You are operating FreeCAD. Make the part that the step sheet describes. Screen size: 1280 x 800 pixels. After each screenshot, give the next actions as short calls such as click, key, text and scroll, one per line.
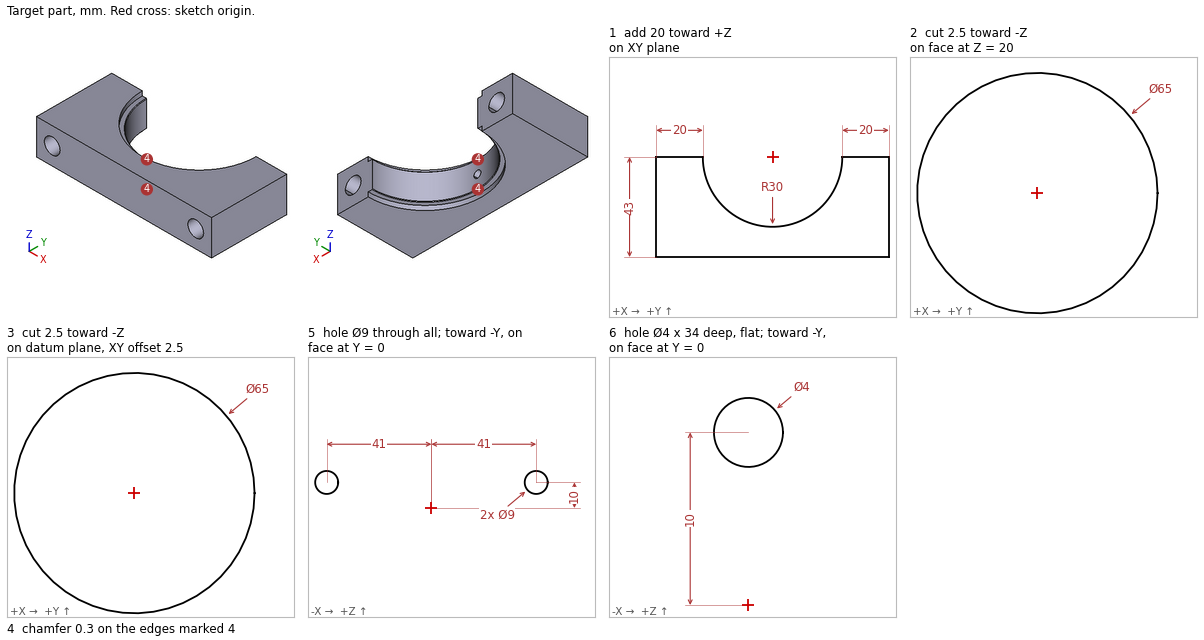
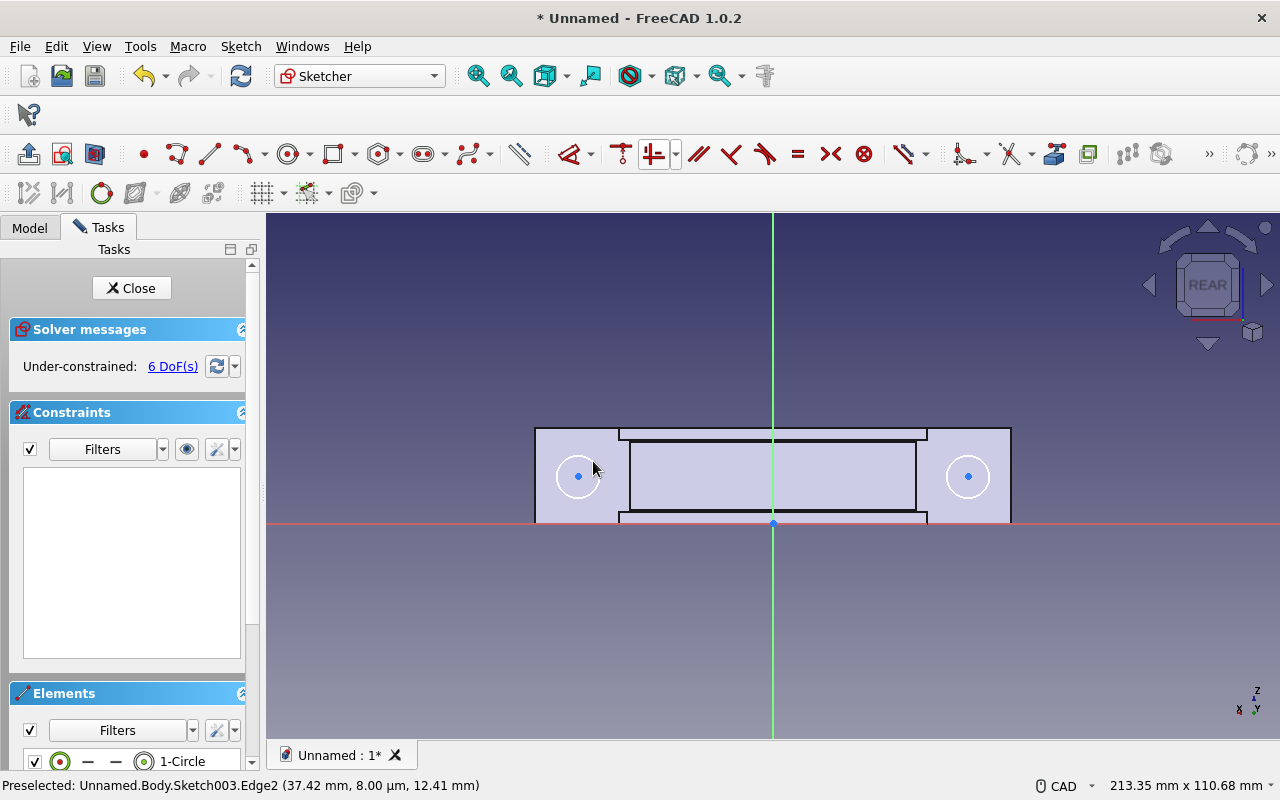
click(983, 462)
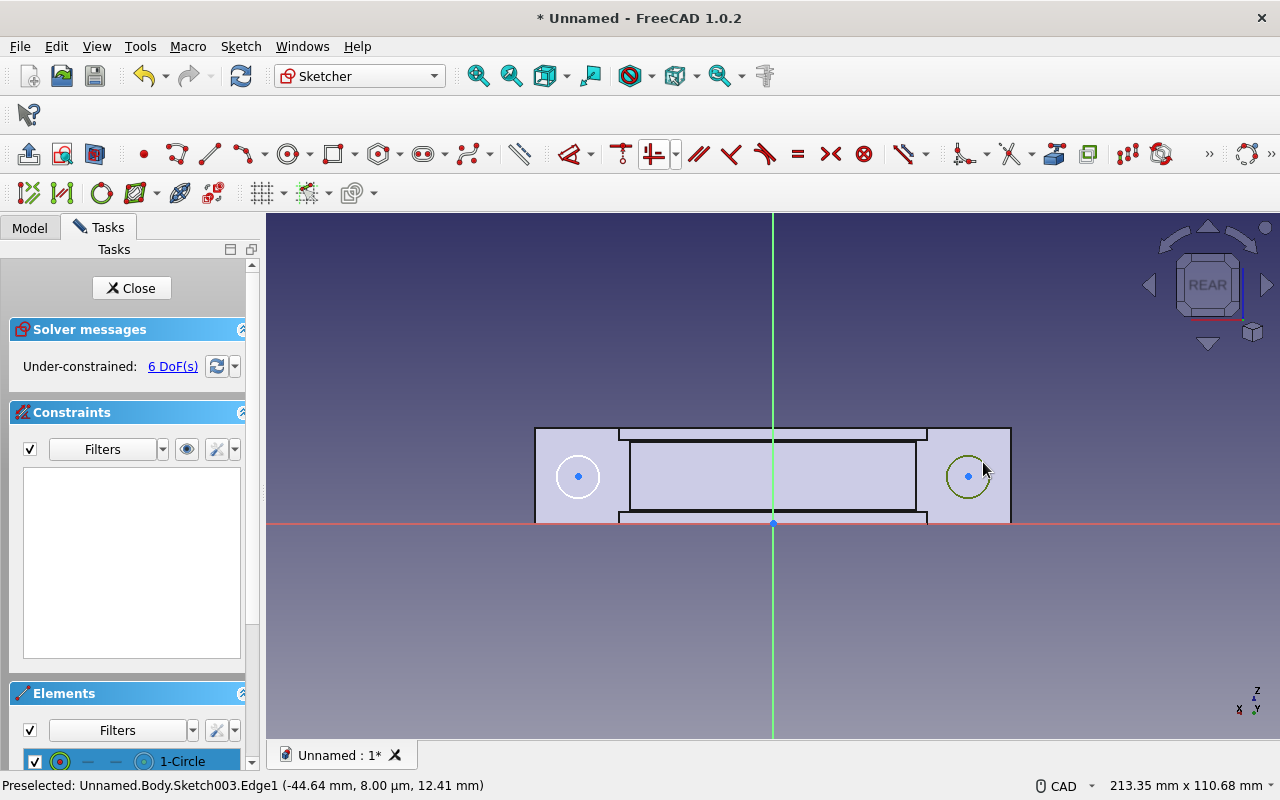
click(593, 462)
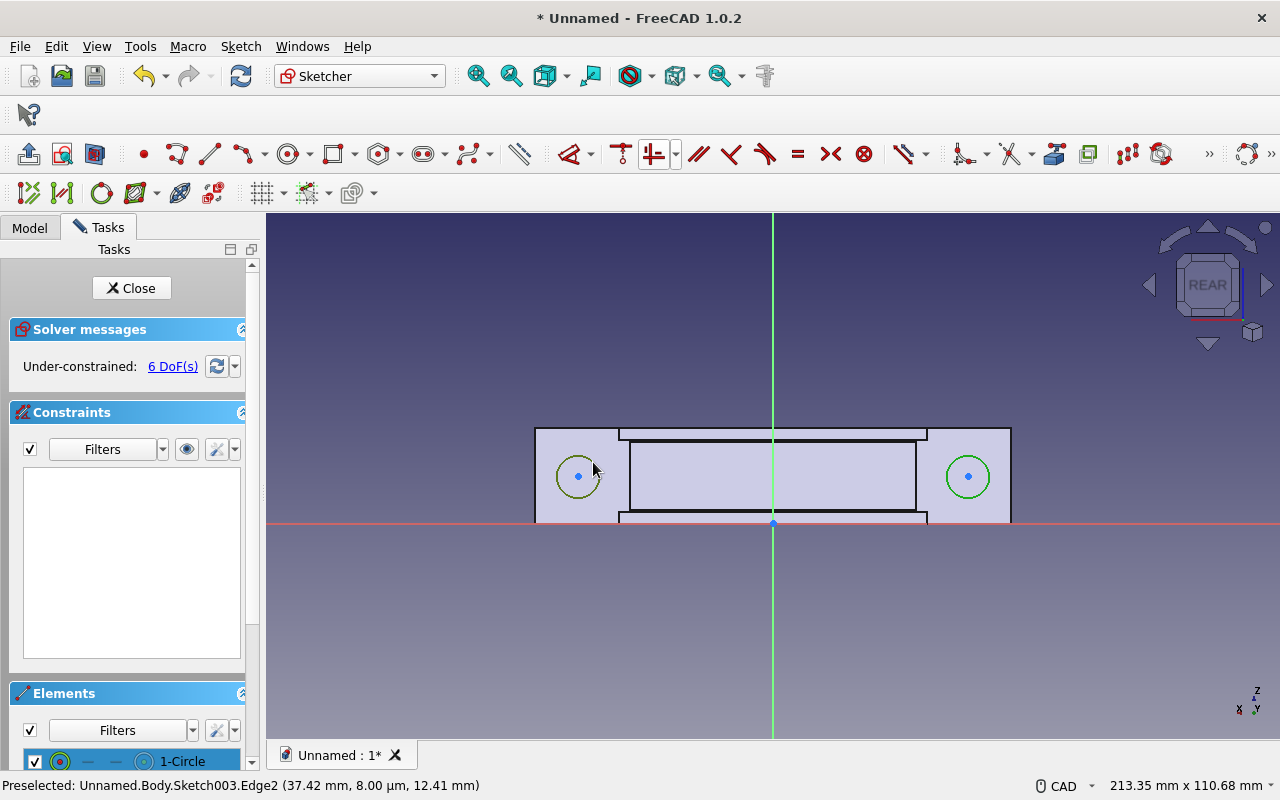
click(798, 154)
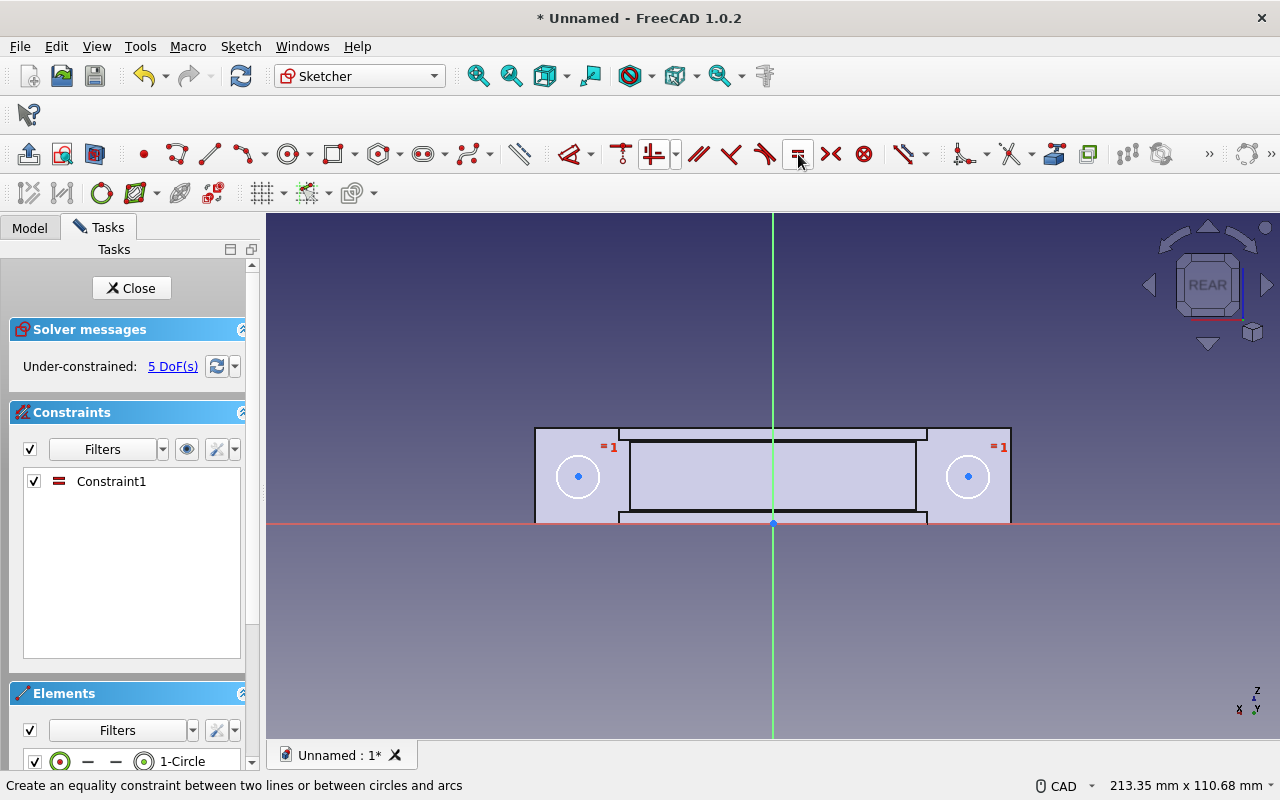
click(968, 477)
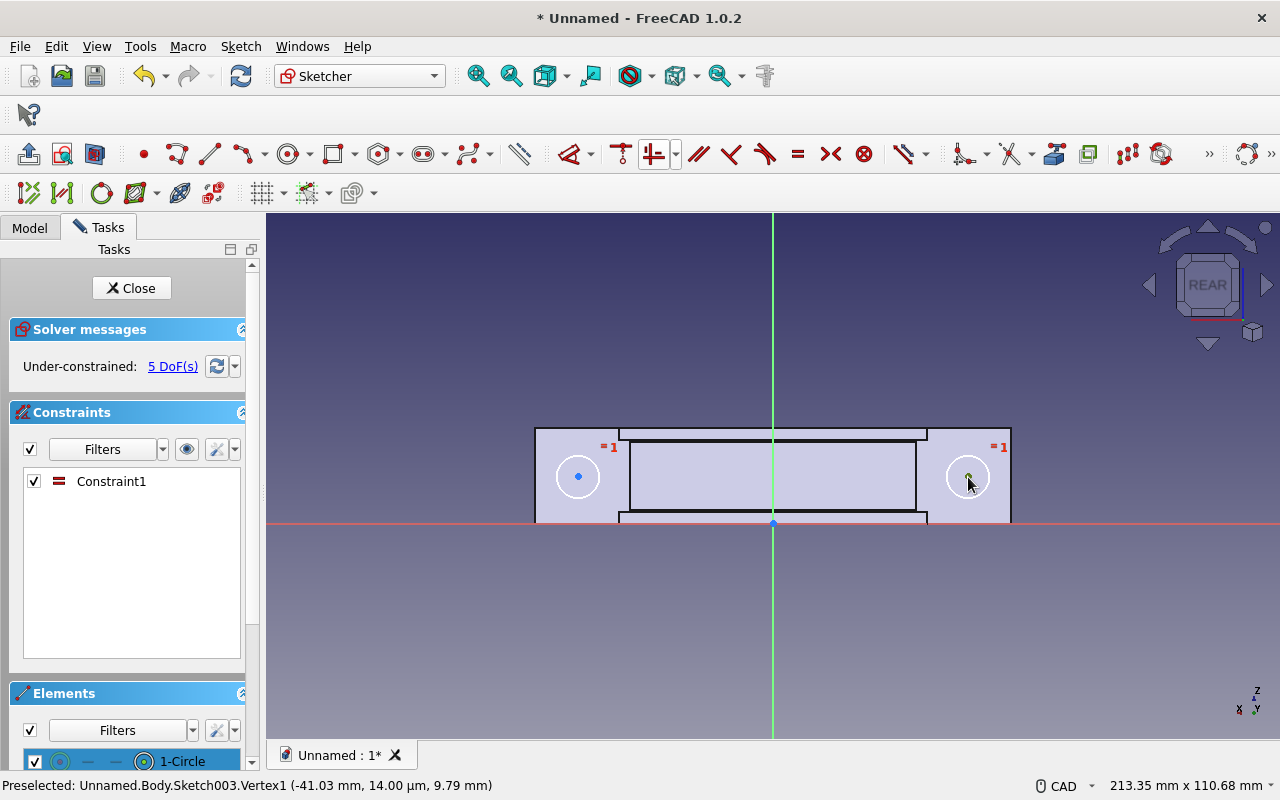
click(578, 477)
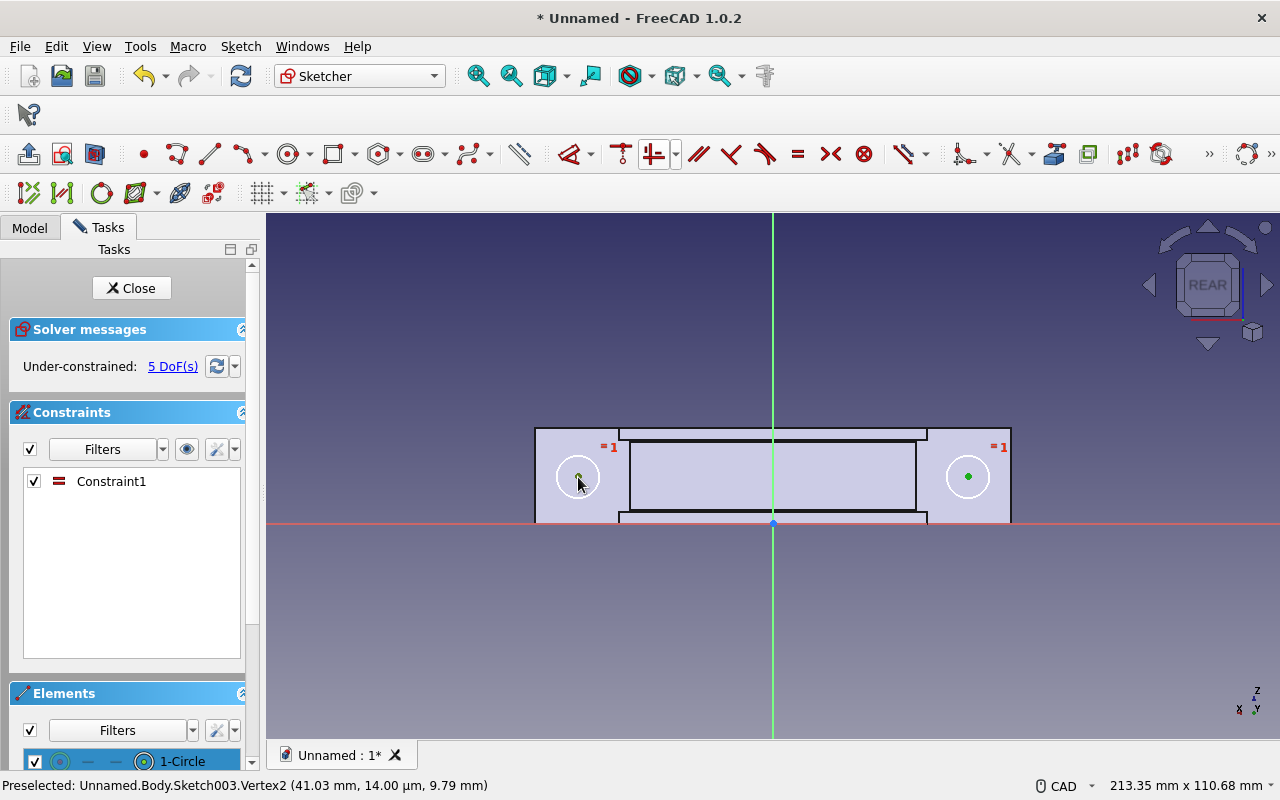
key(h)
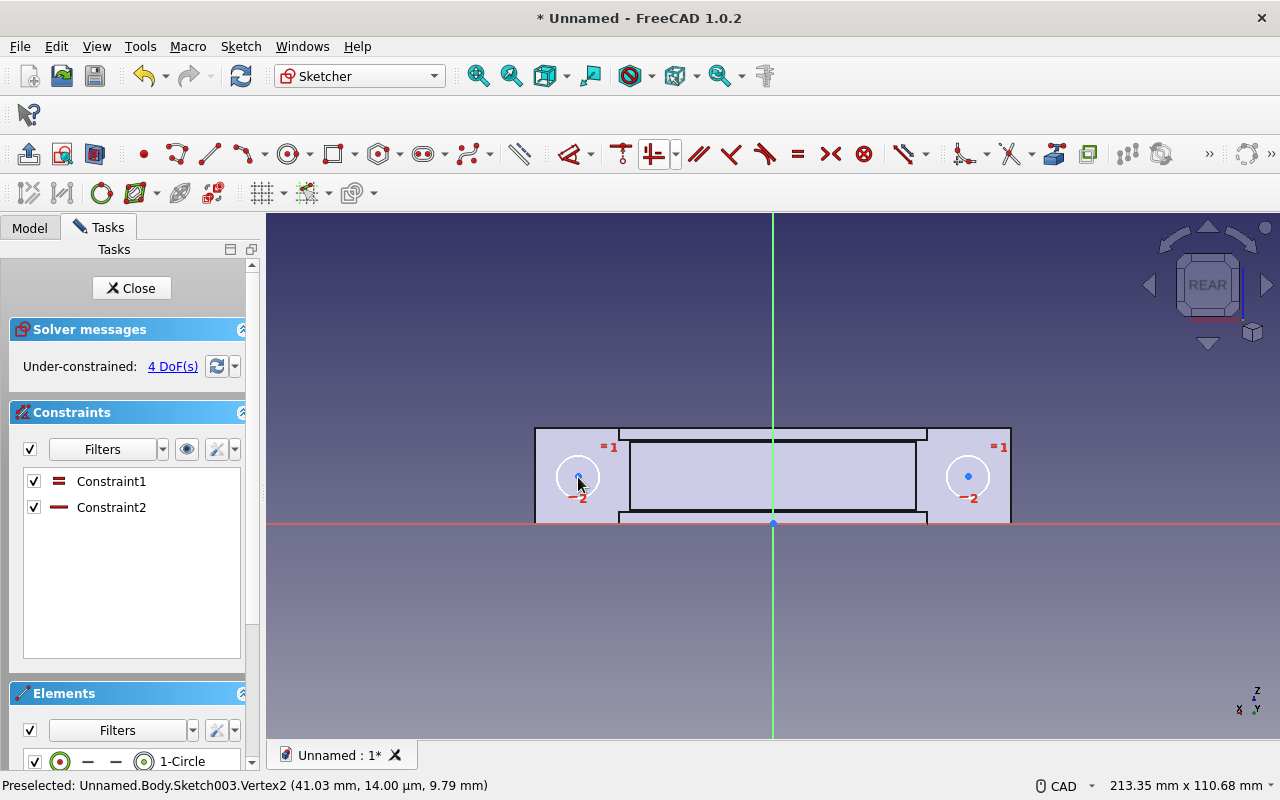
click(568, 154)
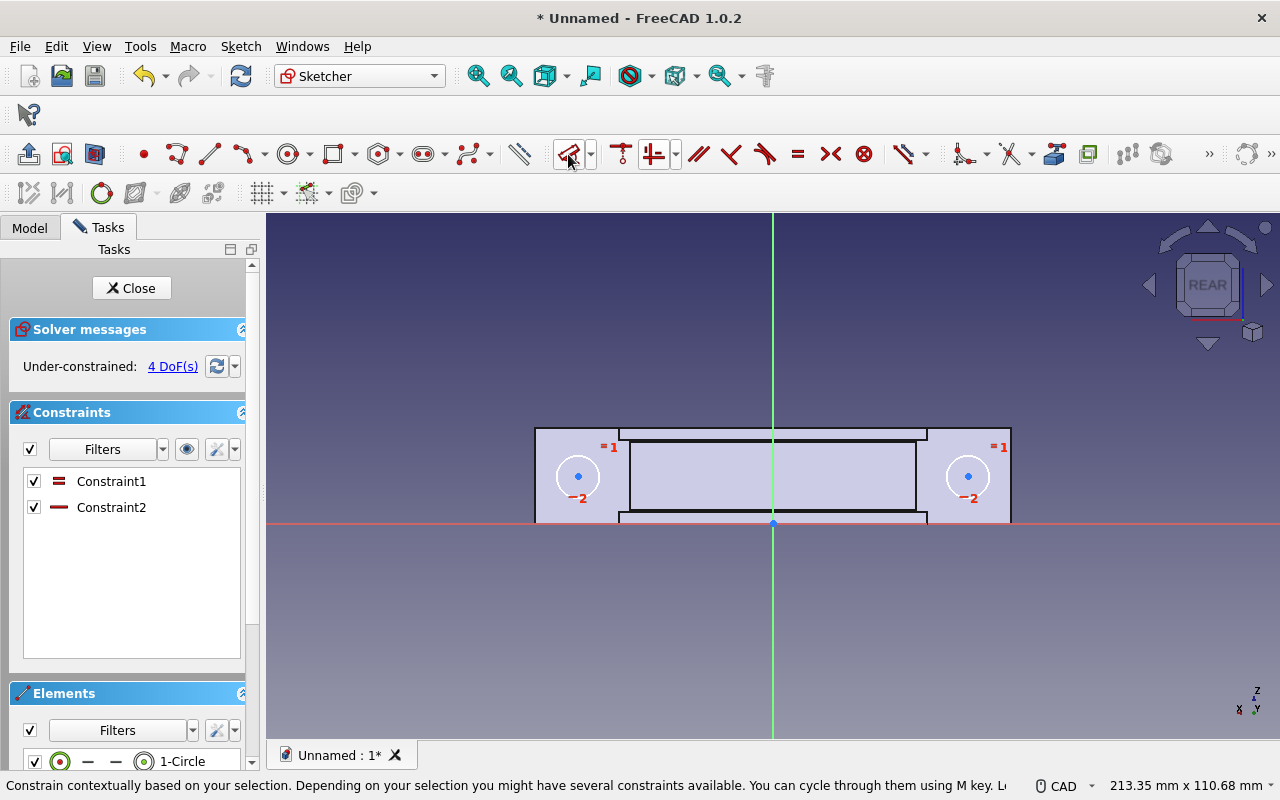
click(983, 462)
click(1006, 439)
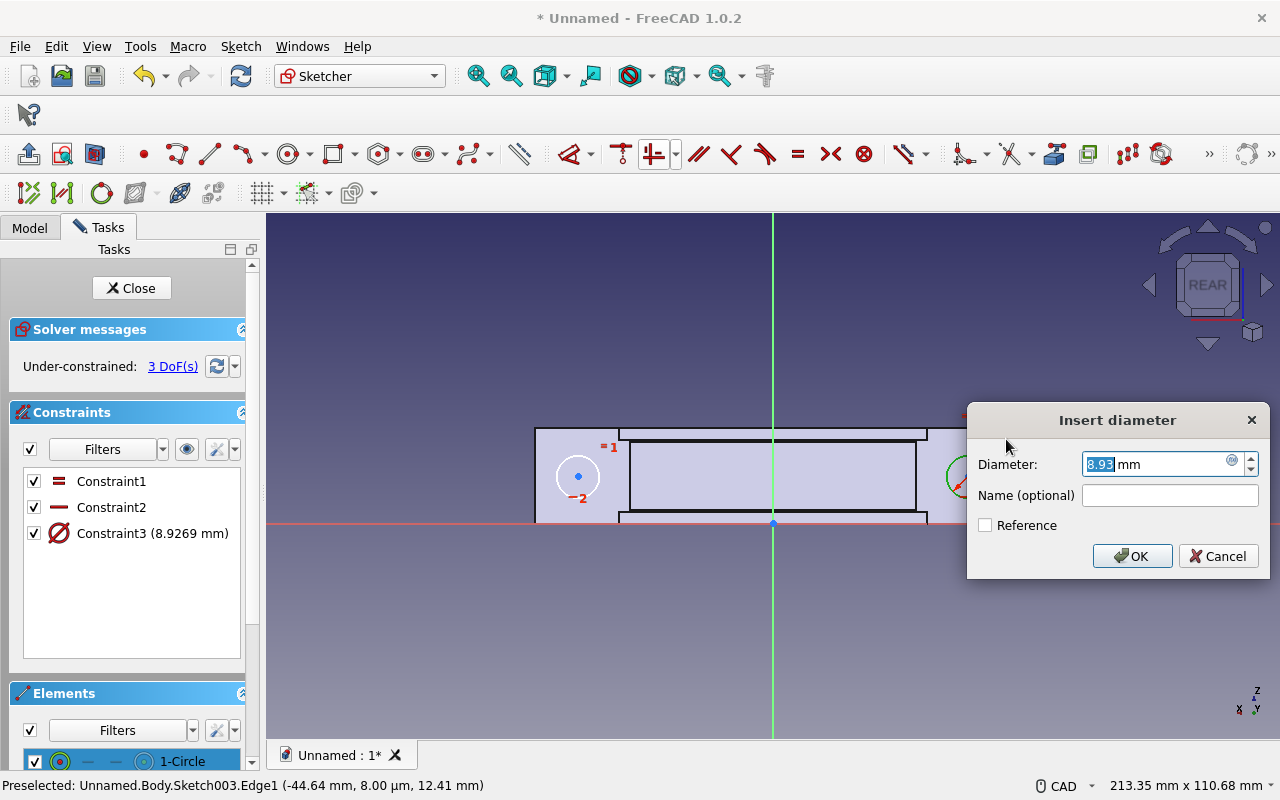
text(9)
key(Return)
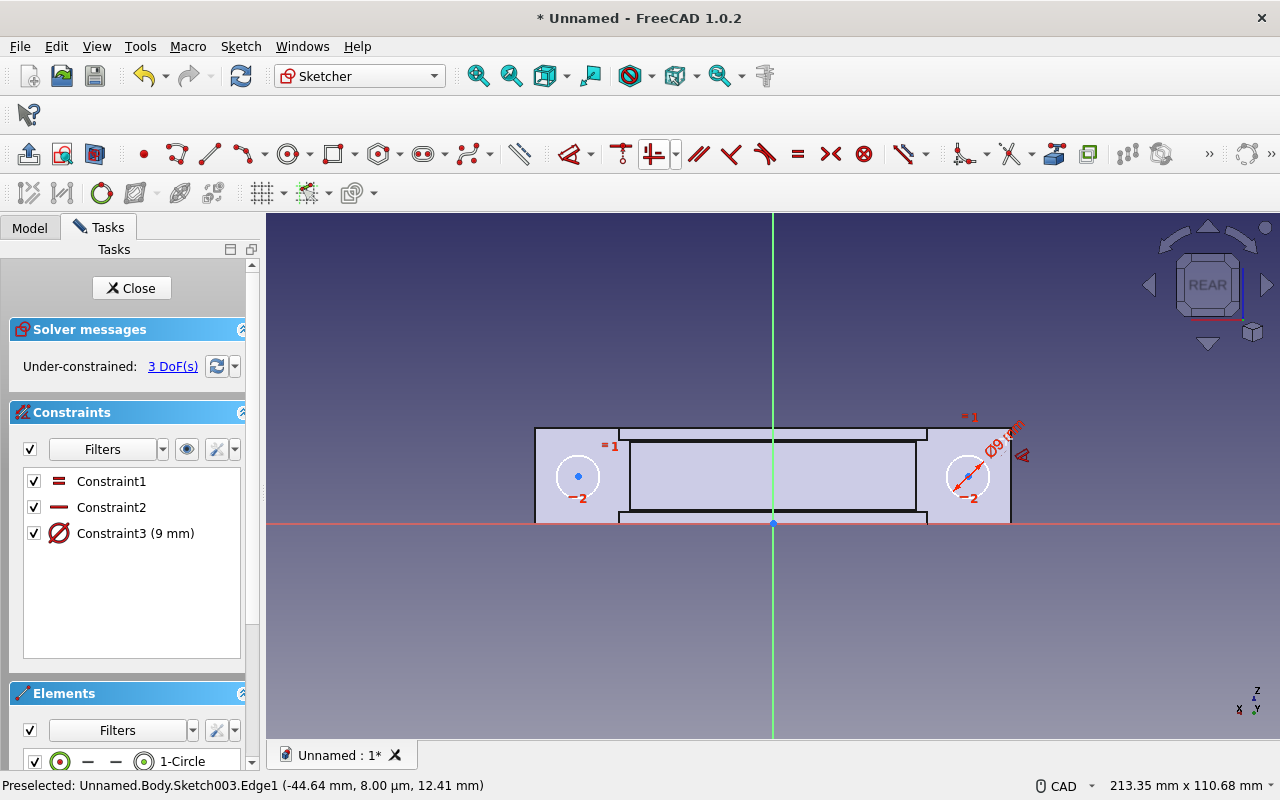
click(968, 477)
click(871, 558)